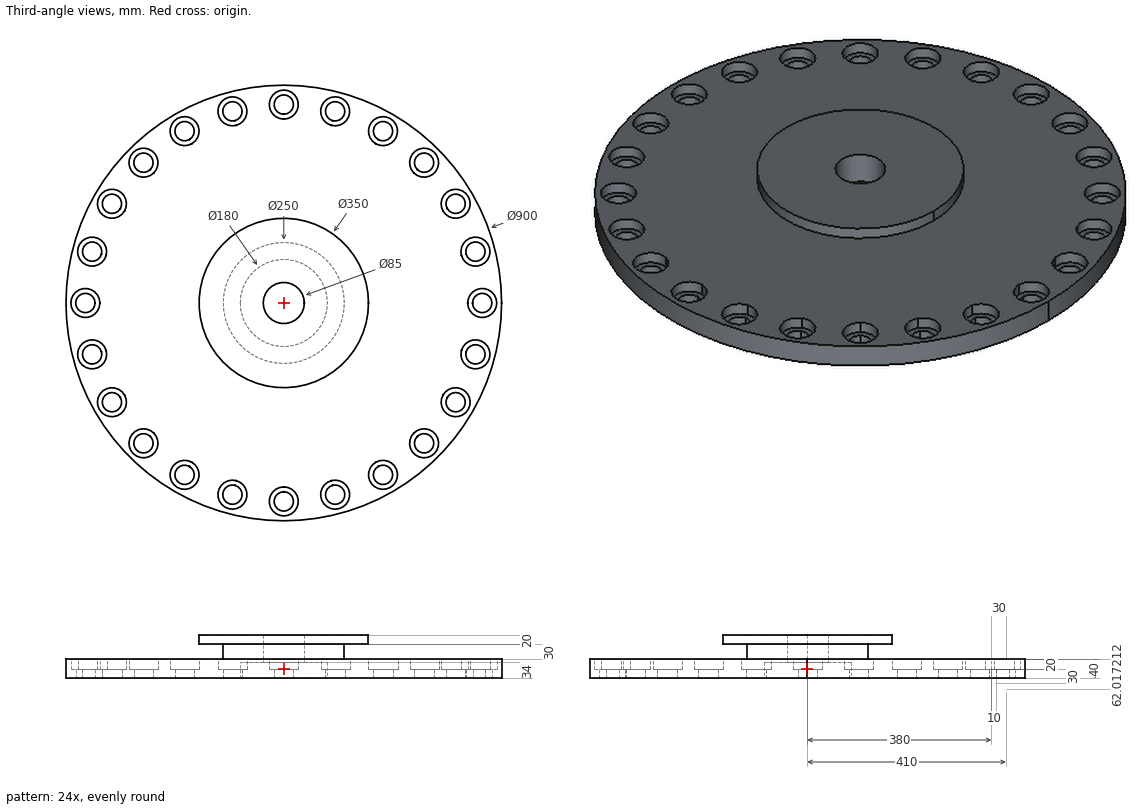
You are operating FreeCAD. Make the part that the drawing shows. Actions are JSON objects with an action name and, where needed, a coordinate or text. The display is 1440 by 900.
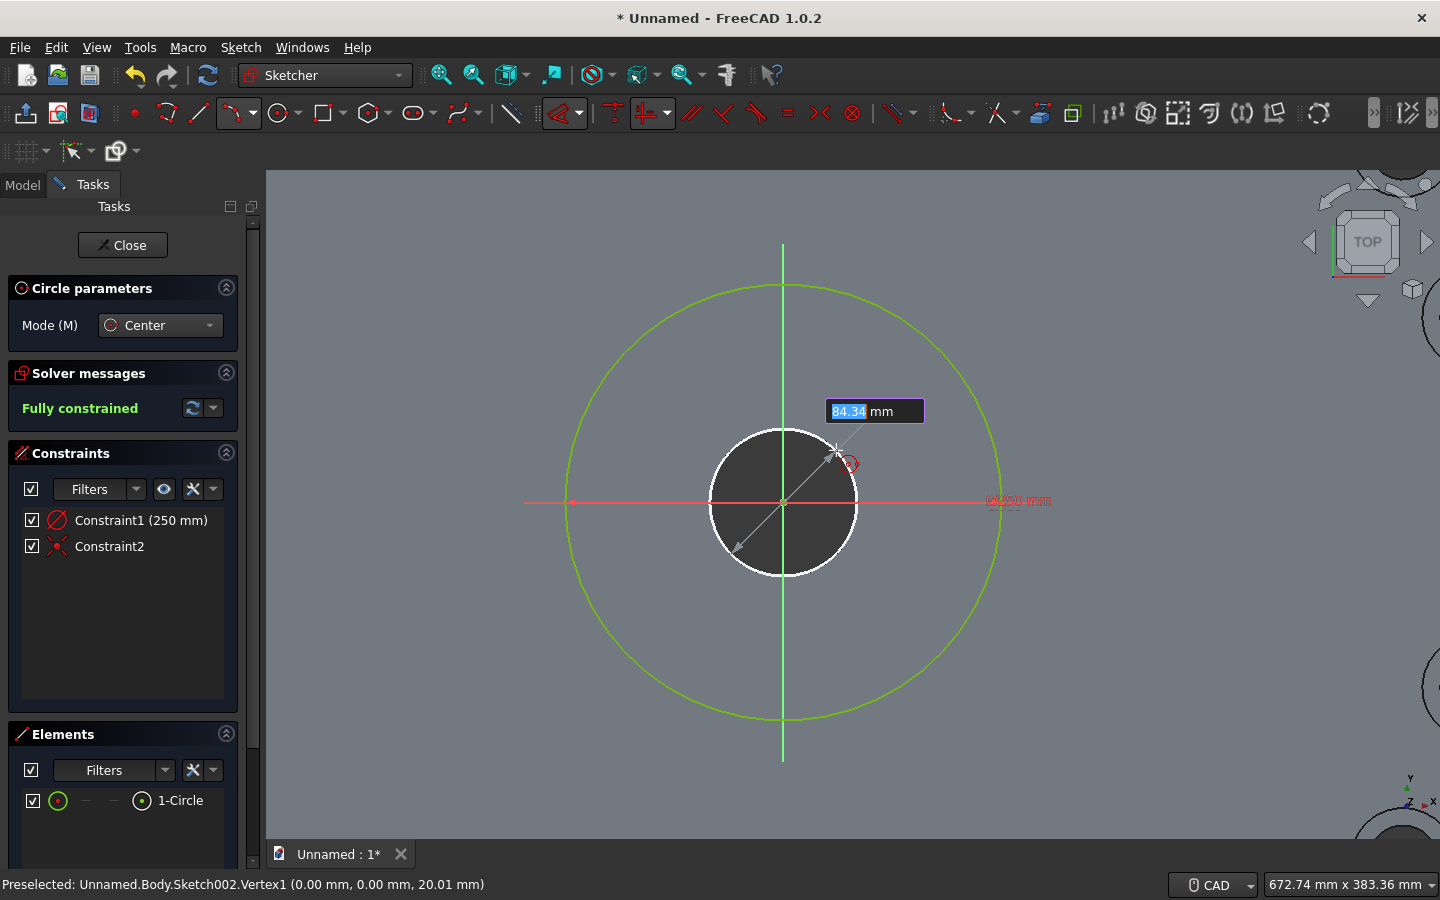
{"action": "type", "text": "85"}
{"action": "key", "text": "Return"}
{"action": "key", "text": "Escape"}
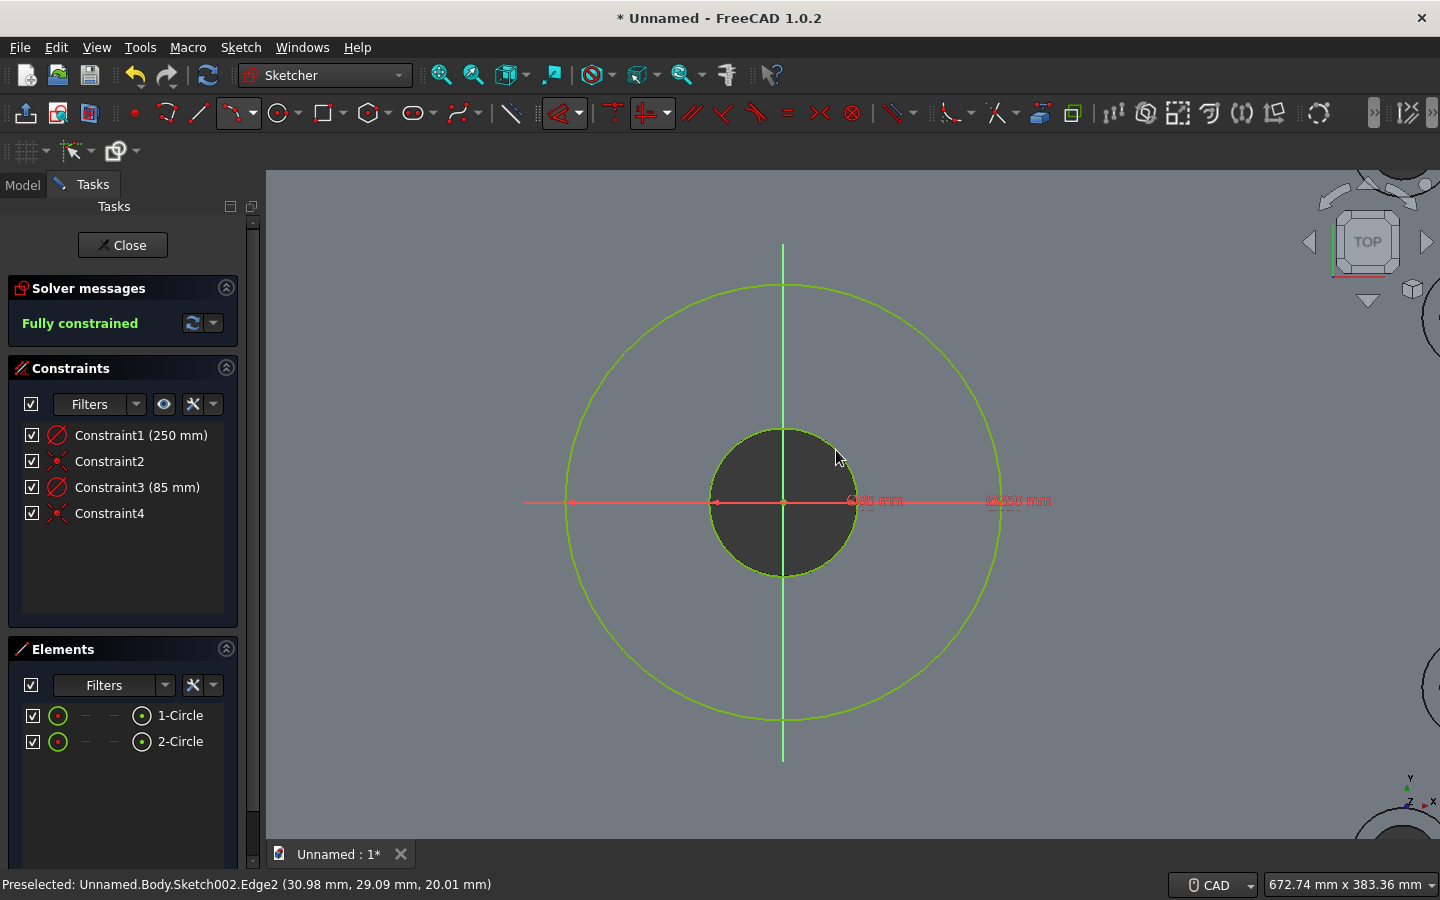
{"action": "left_click", "coordinate": [123, 245]}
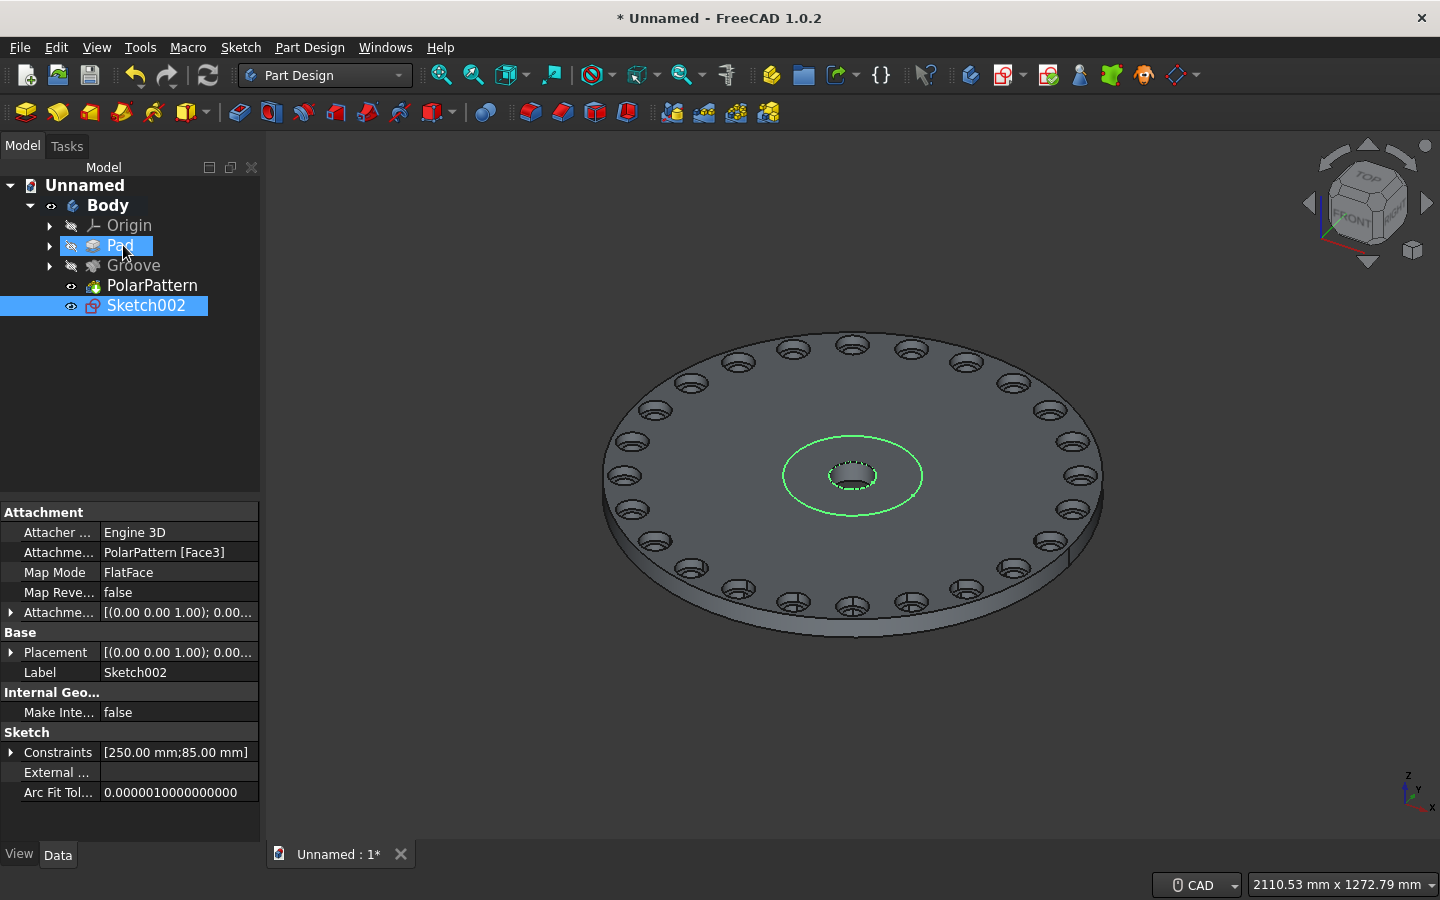
{"action": "left_click", "coordinate": [26, 112]}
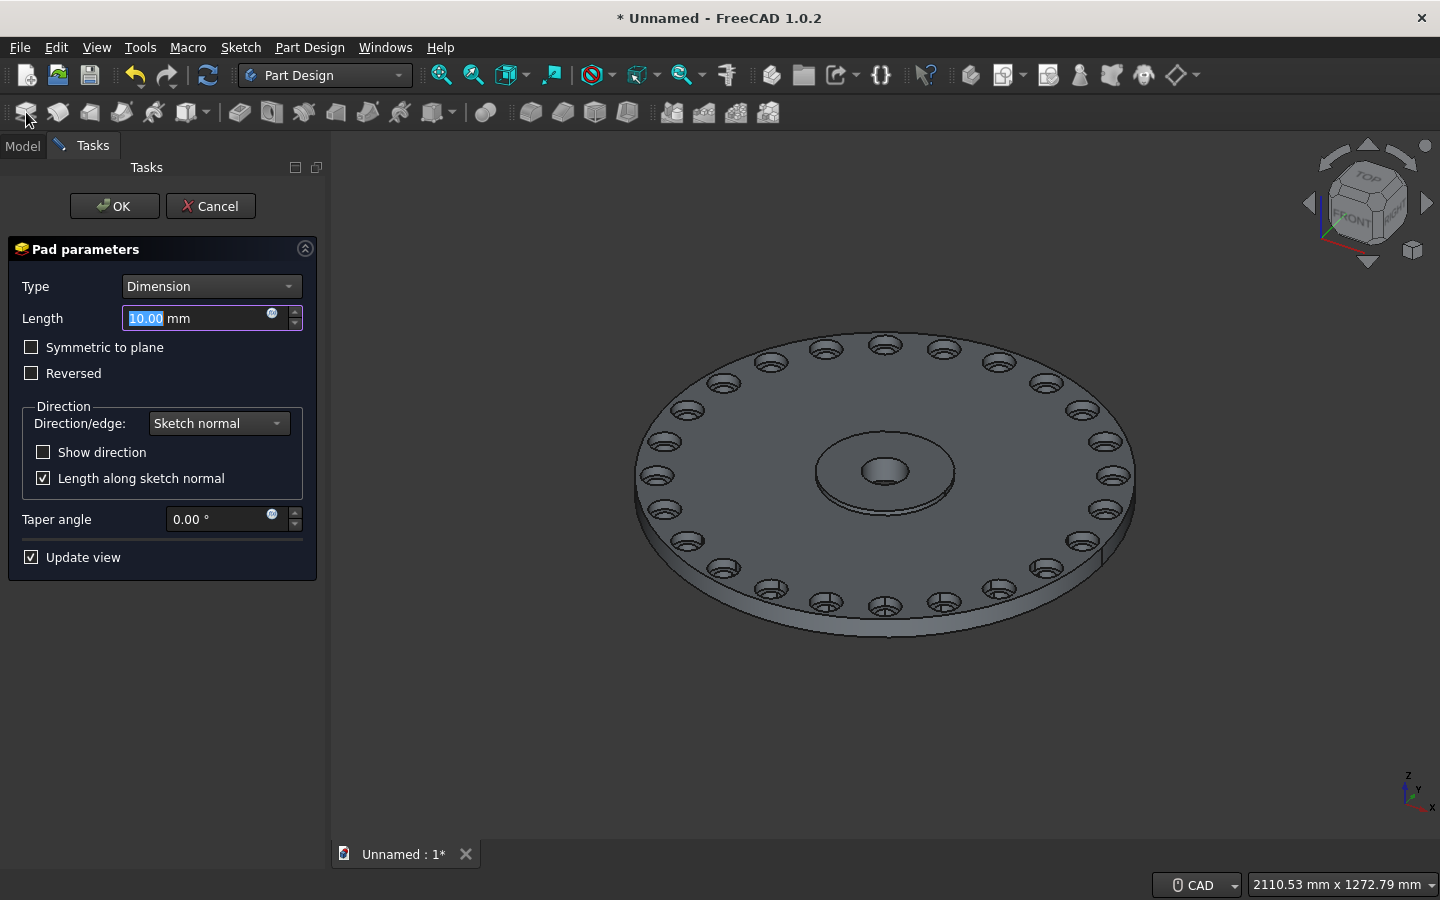
{"action": "type", "text": "30"}
{"action": "key", "text": "Tab"}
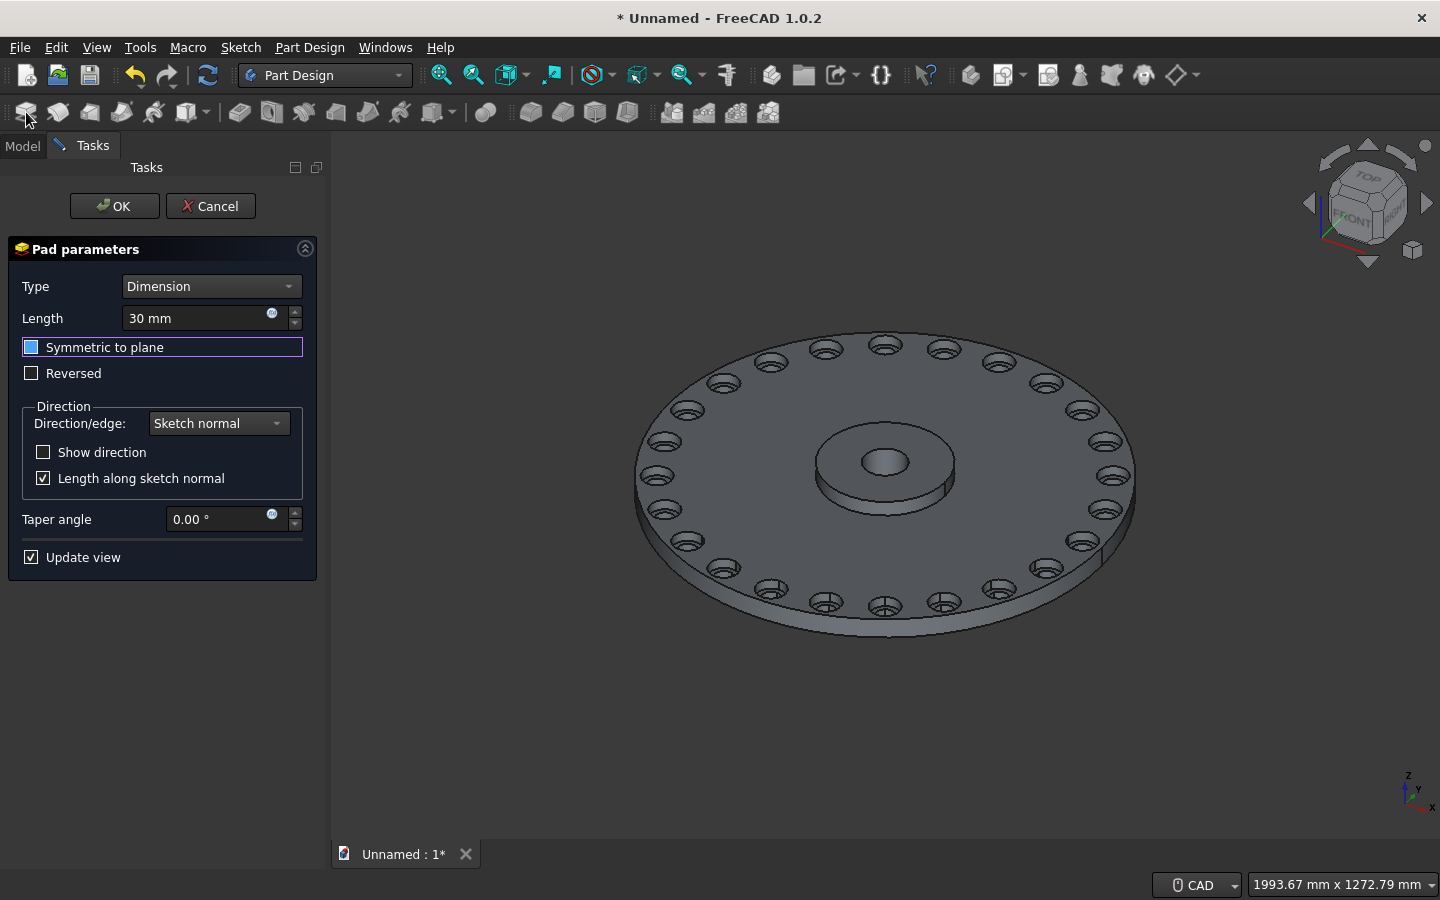
{"action": "left_click", "coordinate": [115, 206]}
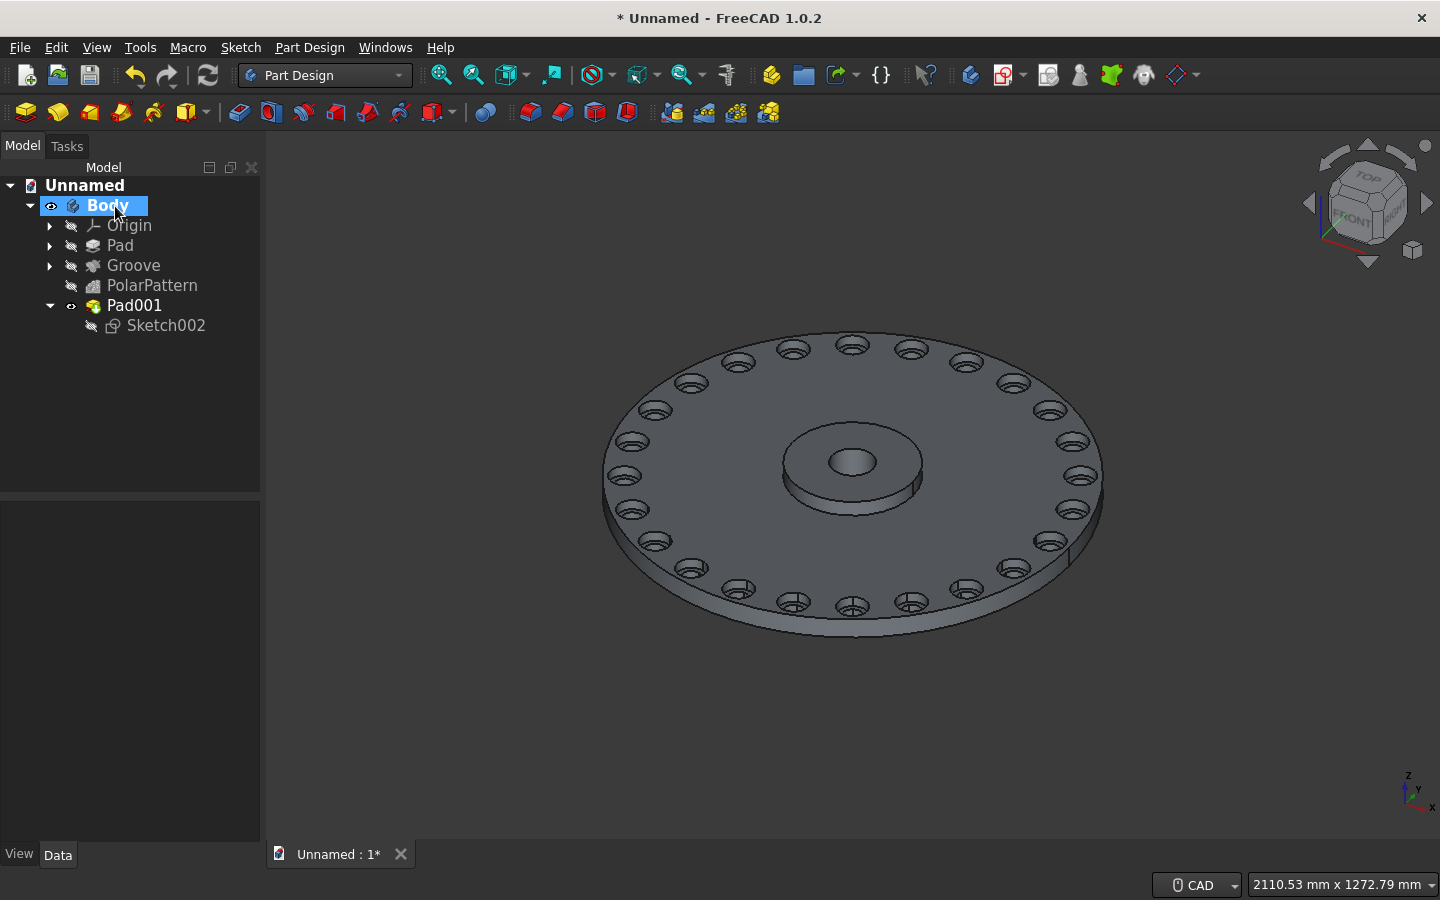
{"action": "left_click", "coordinate": [816, 475]}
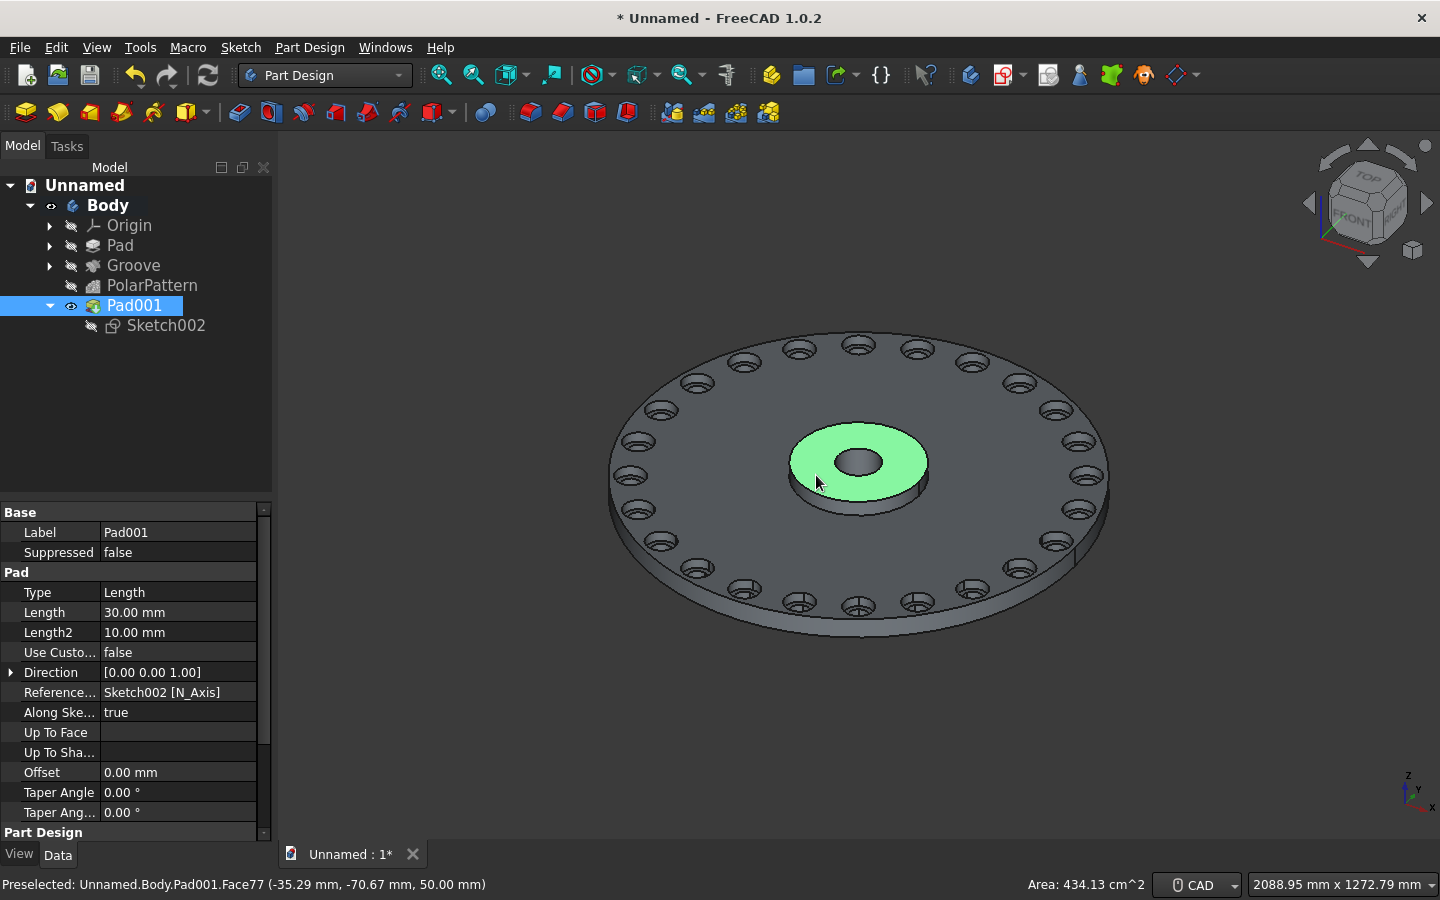
{"action": "left_click", "coordinate": [1004, 76]}